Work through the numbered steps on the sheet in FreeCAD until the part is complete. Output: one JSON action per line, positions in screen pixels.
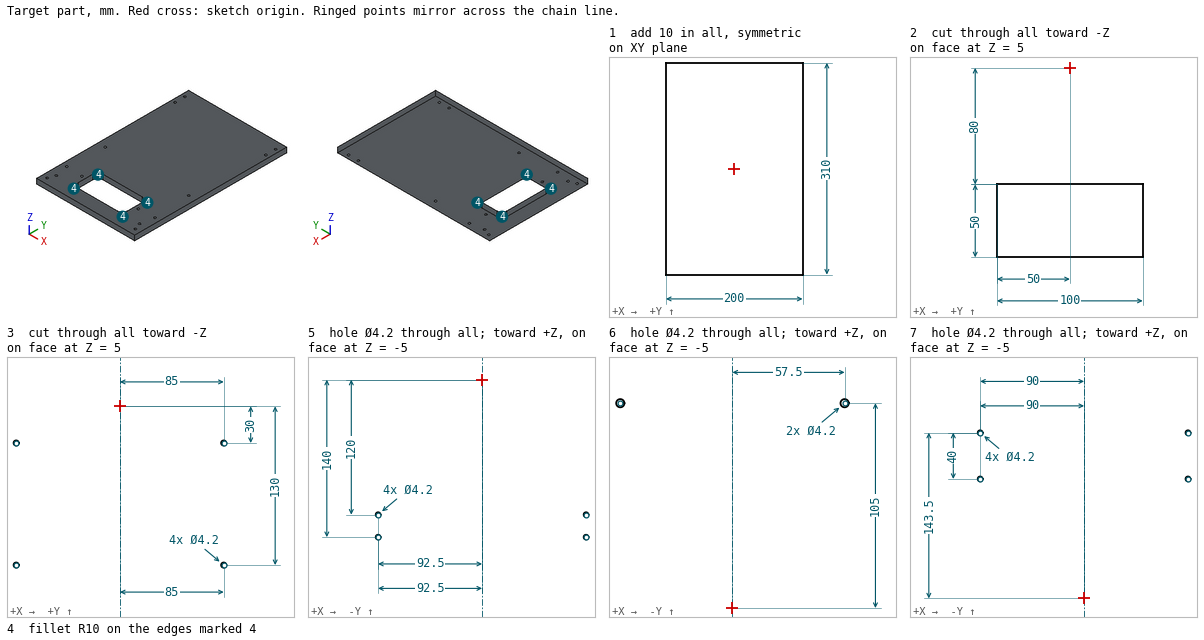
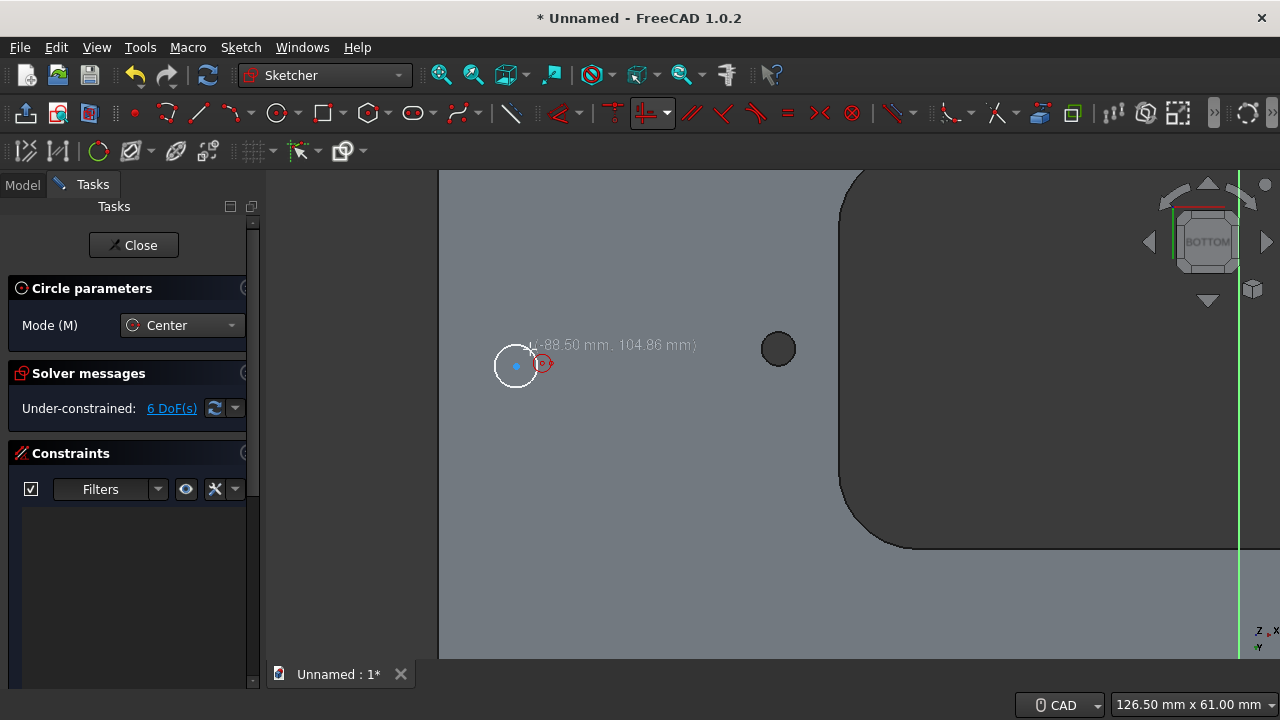
{"action": "scroll", "coordinate": [529, 351], "scroll_direction": "down", "scroll_amount": 7}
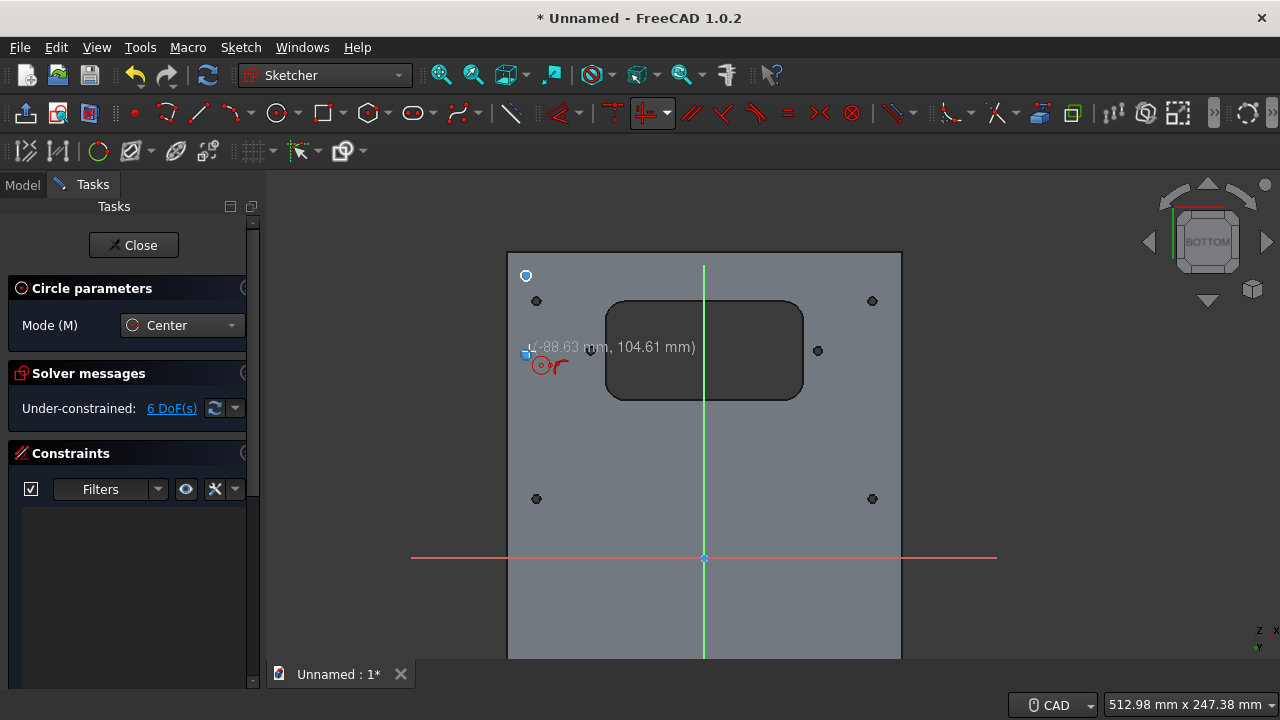
{"action": "scroll", "coordinate": [882, 354], "scroll_direction": "up", "scroll_amount": 9}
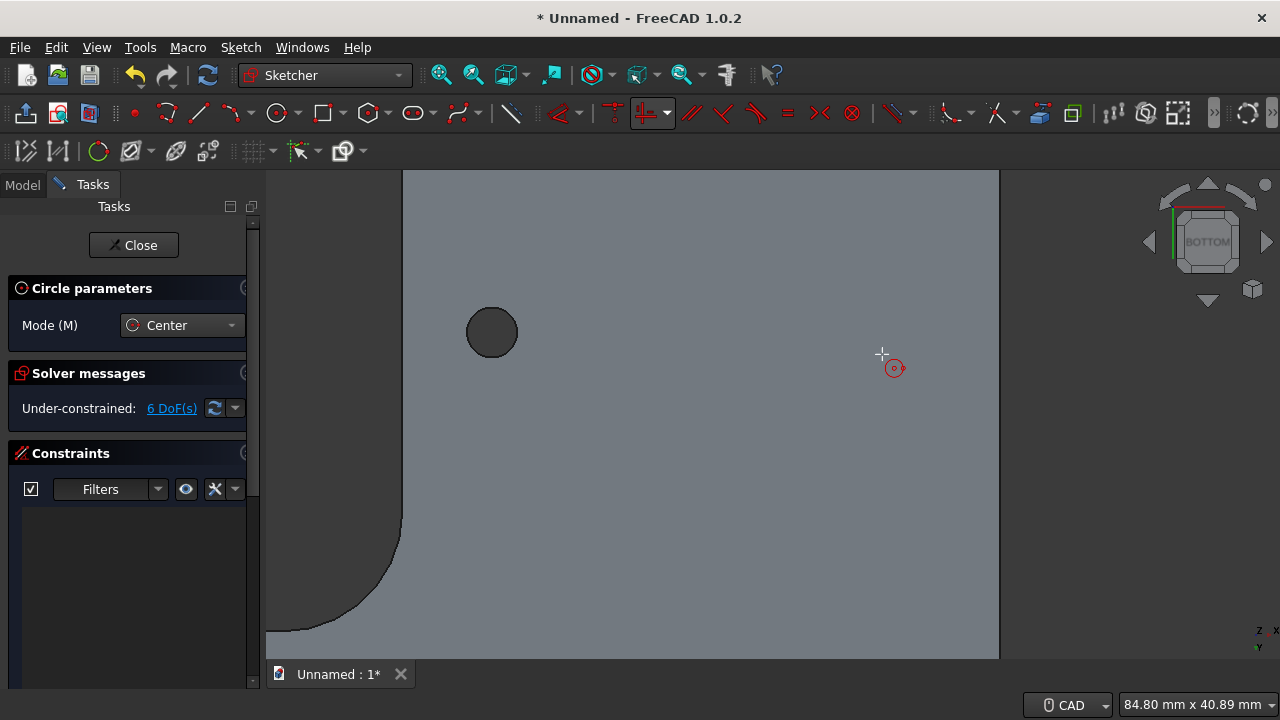
{"action": "scroll", "coordinate": [883, 354], "scroll_direction": "down", "scroll_amount": 9}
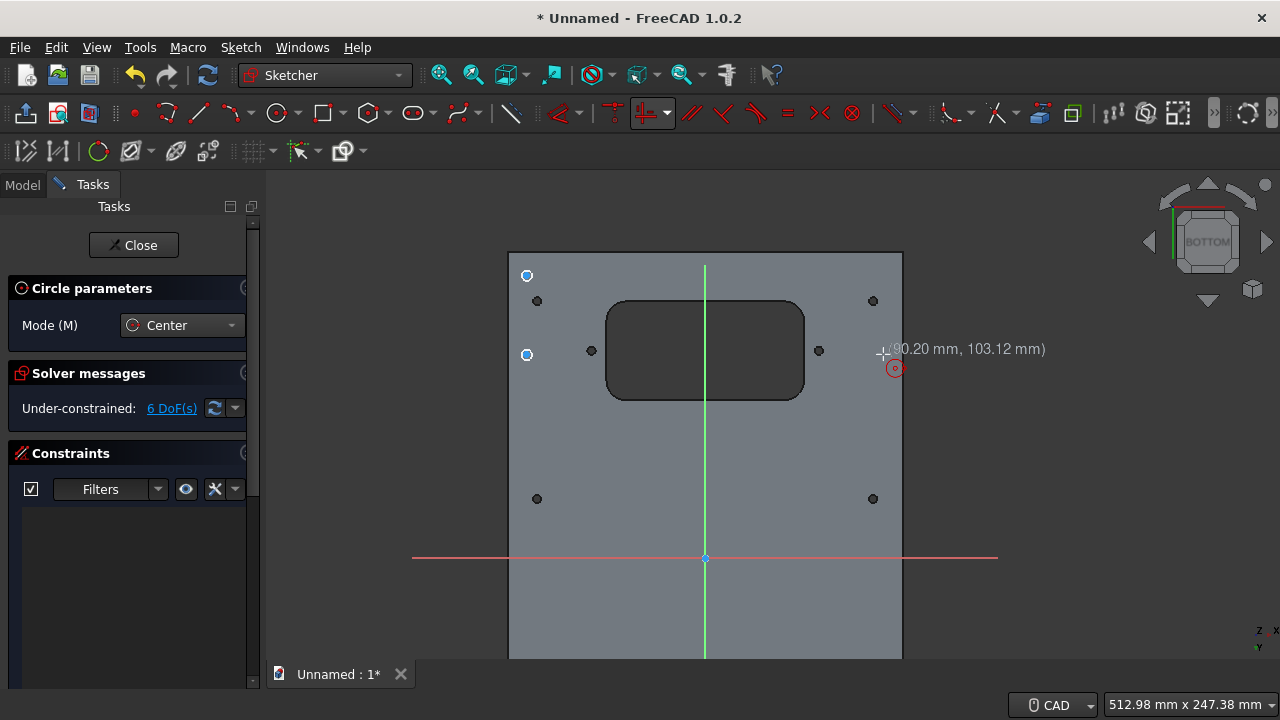
{"action": "left_click", "coordinate": [883, 354]}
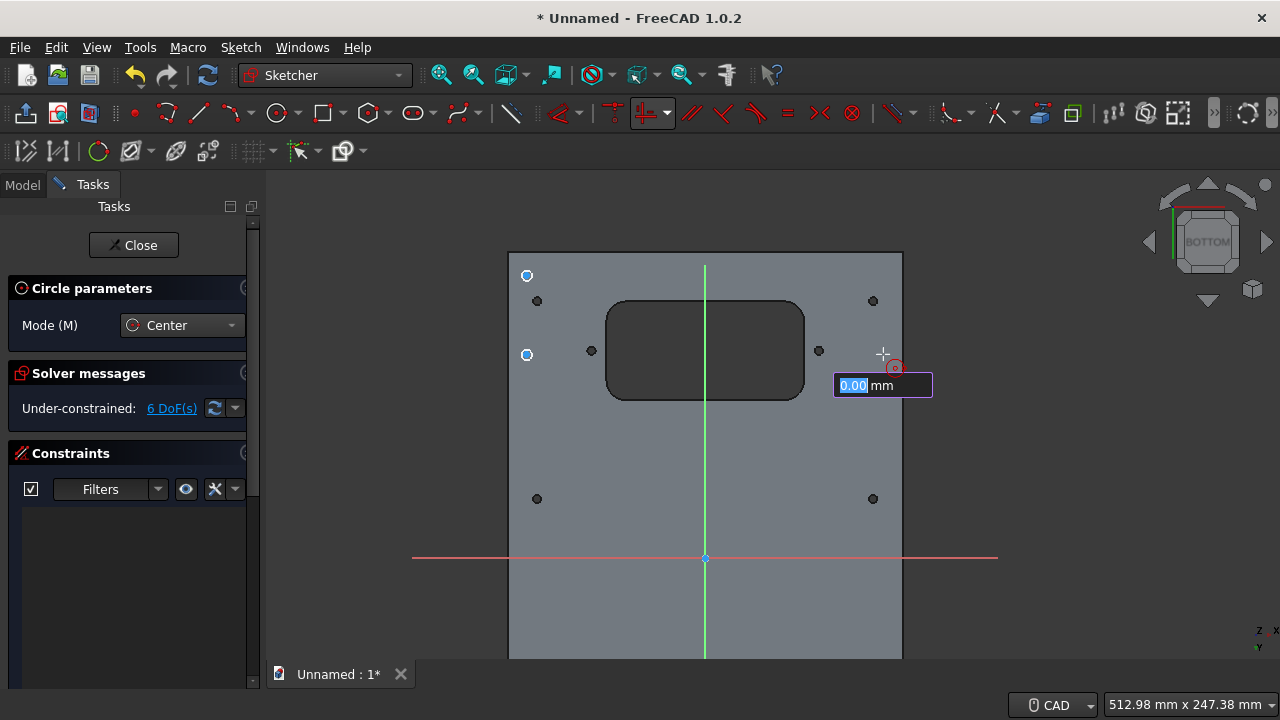
{"action": "scroll", "coordinate": [886, 351], "scroll_direction": "up", "scroll_amount": 7}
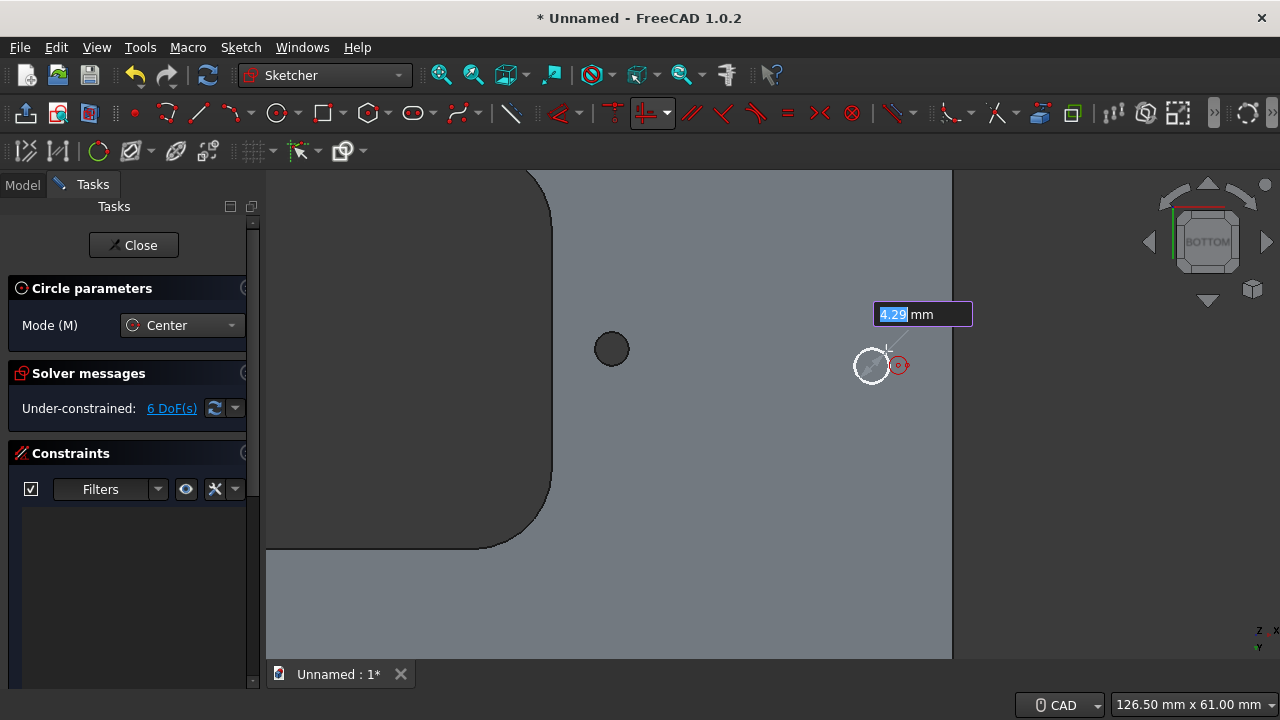
{"action": "left_click", "coordinate": [884, 349]}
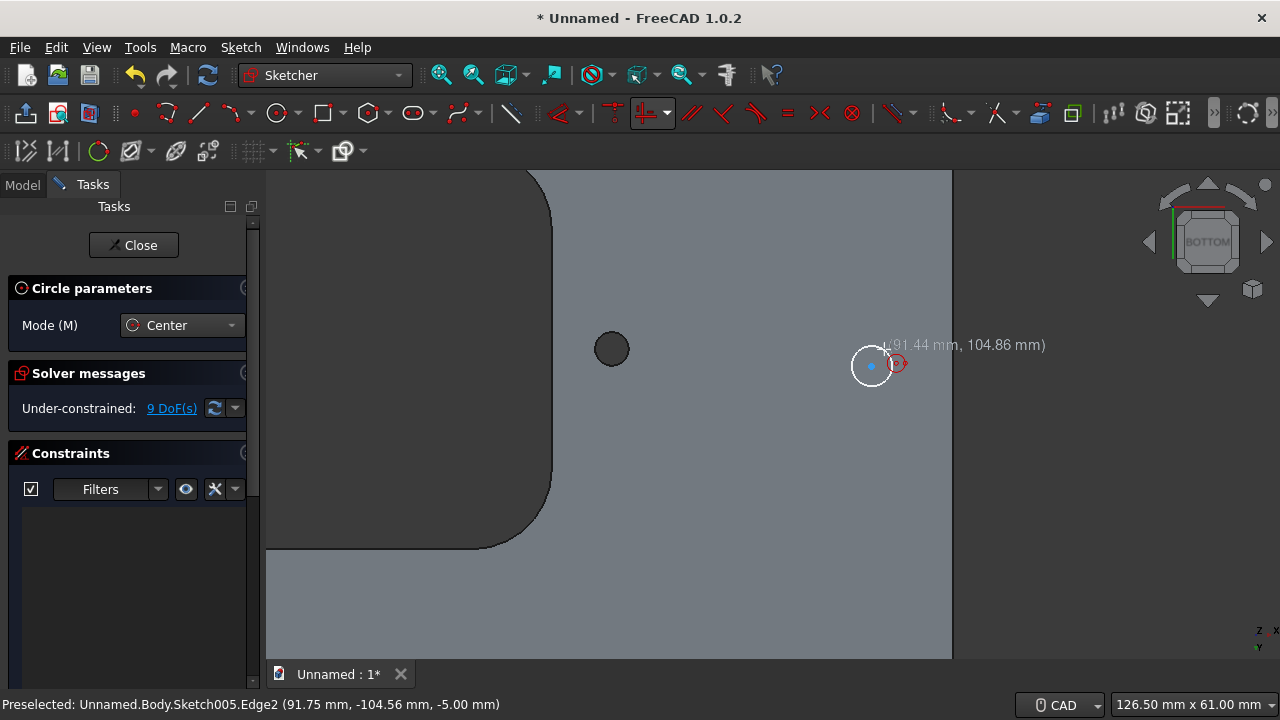
{"action": "scroll", "coordinate": [886, 351], "scroll_direction": "down", "scroll_amount": 7}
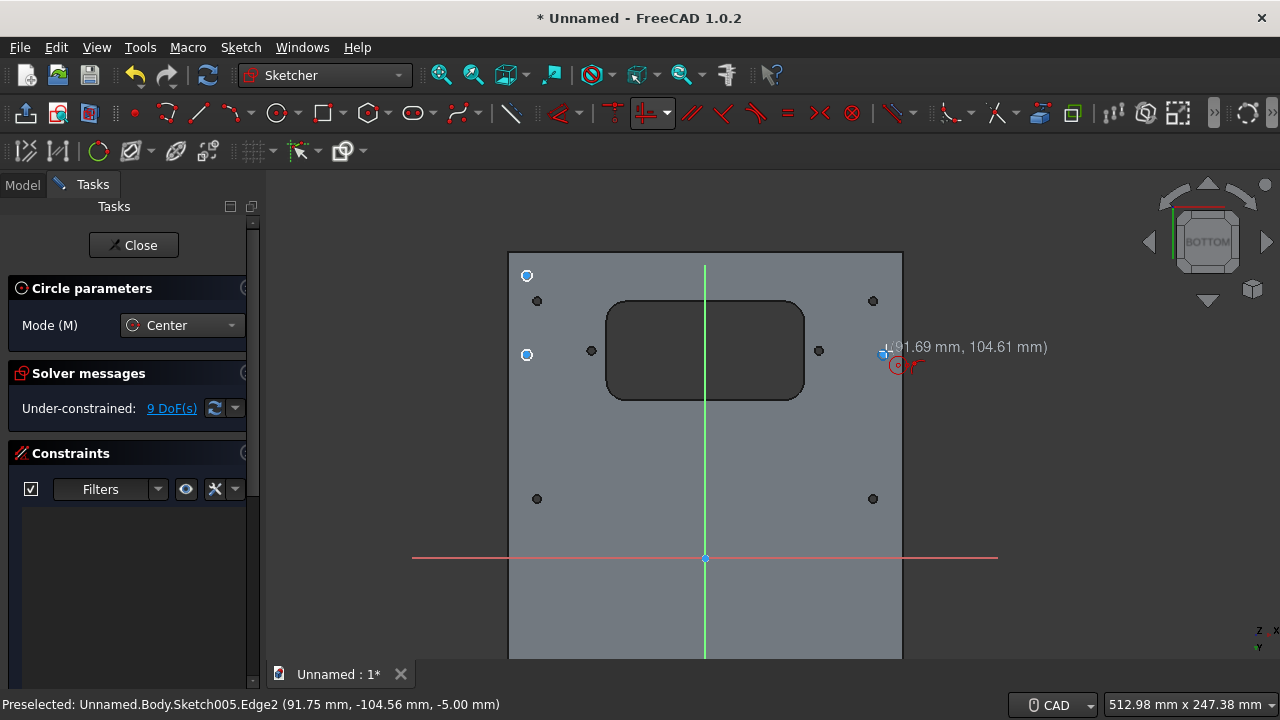
{"action": "scroll", "coordinate": [883, 275], "scroll_direction": "up", "scroll_amount": 9}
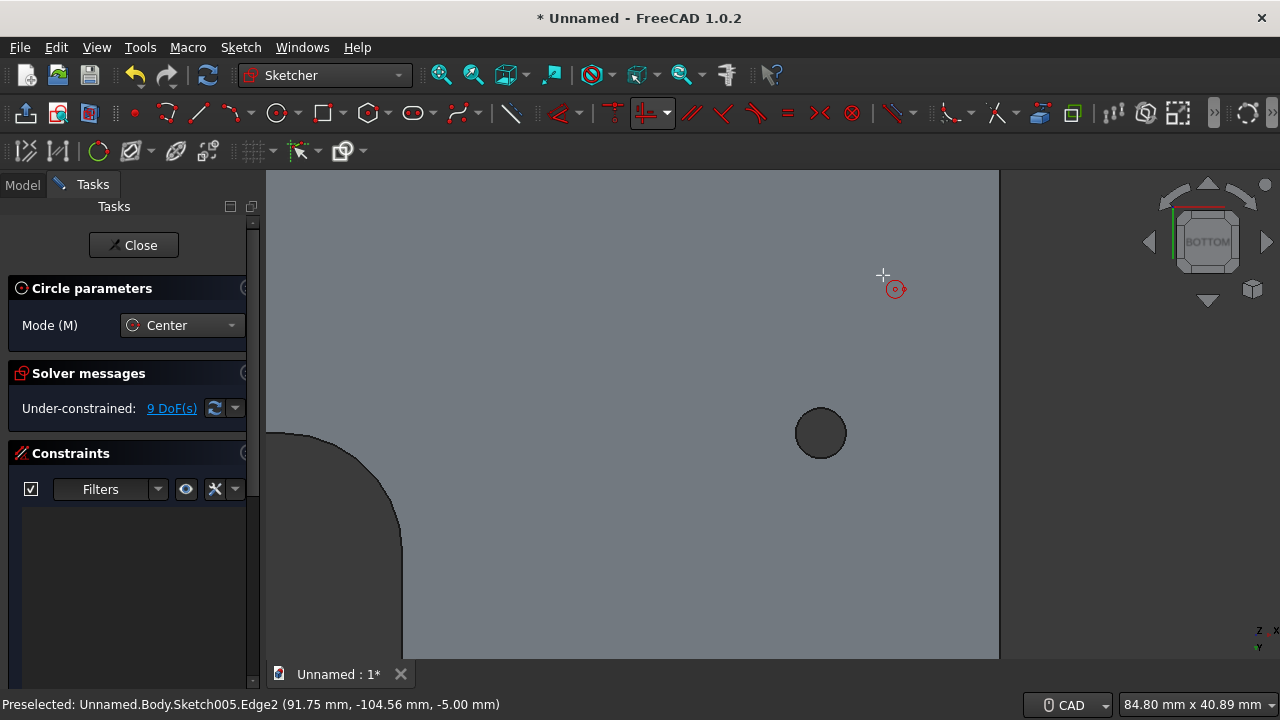
{"action": "scroll", "coordinate": [883, 275], "scroll_direction": "down", "scroll_amount": 9}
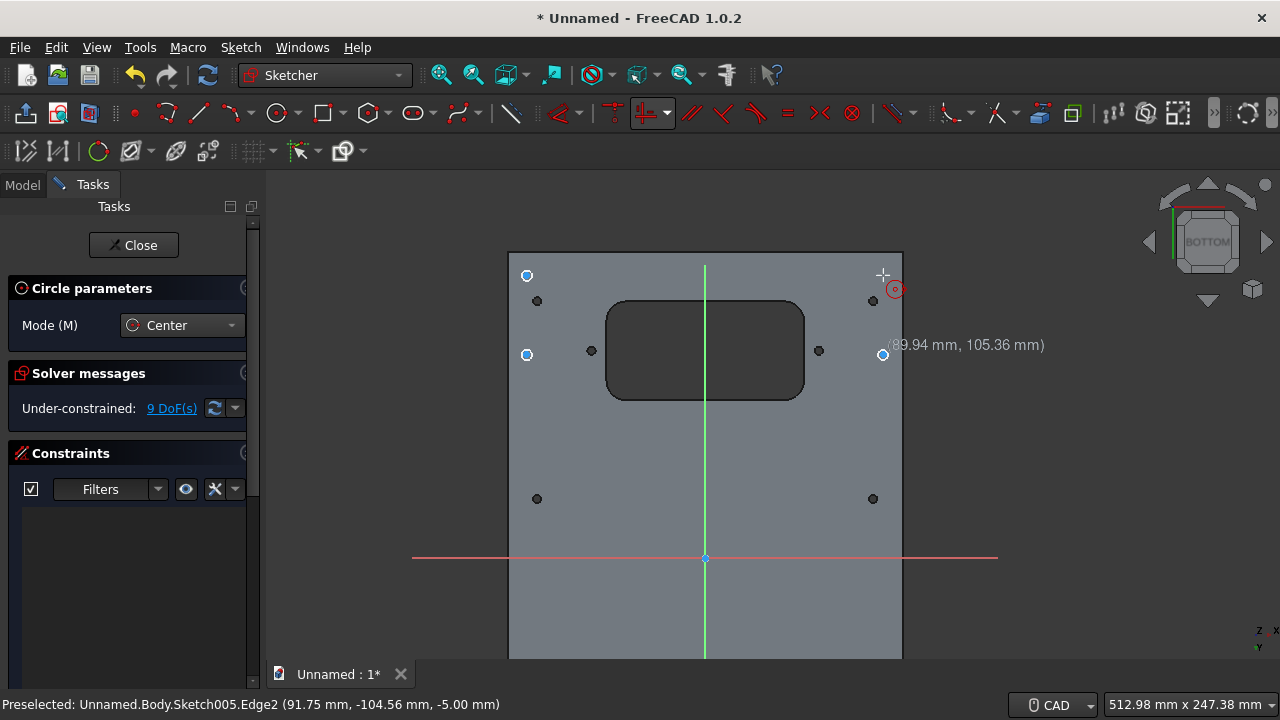
{"action": "left_click", "coordinate": [883, 275]}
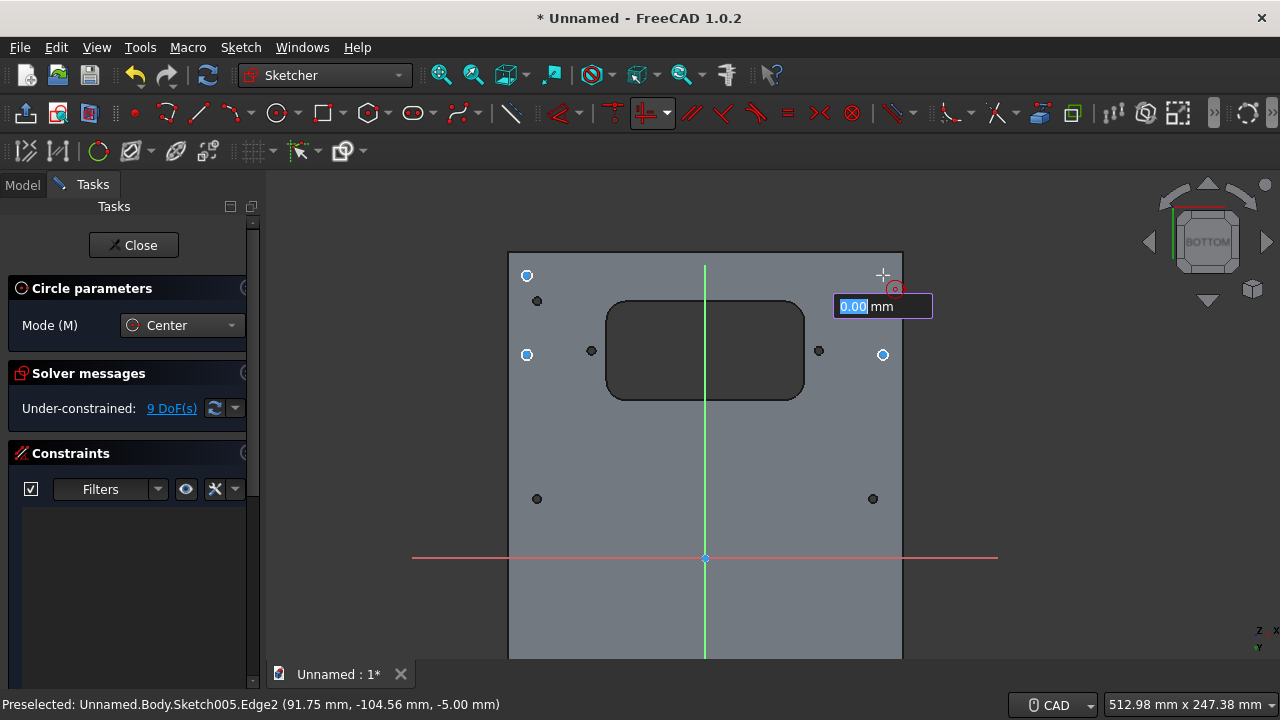
{"action": "scroll", "coordinate": [886, 272], "scroll_direction": "up", "scroll_amount": 7}